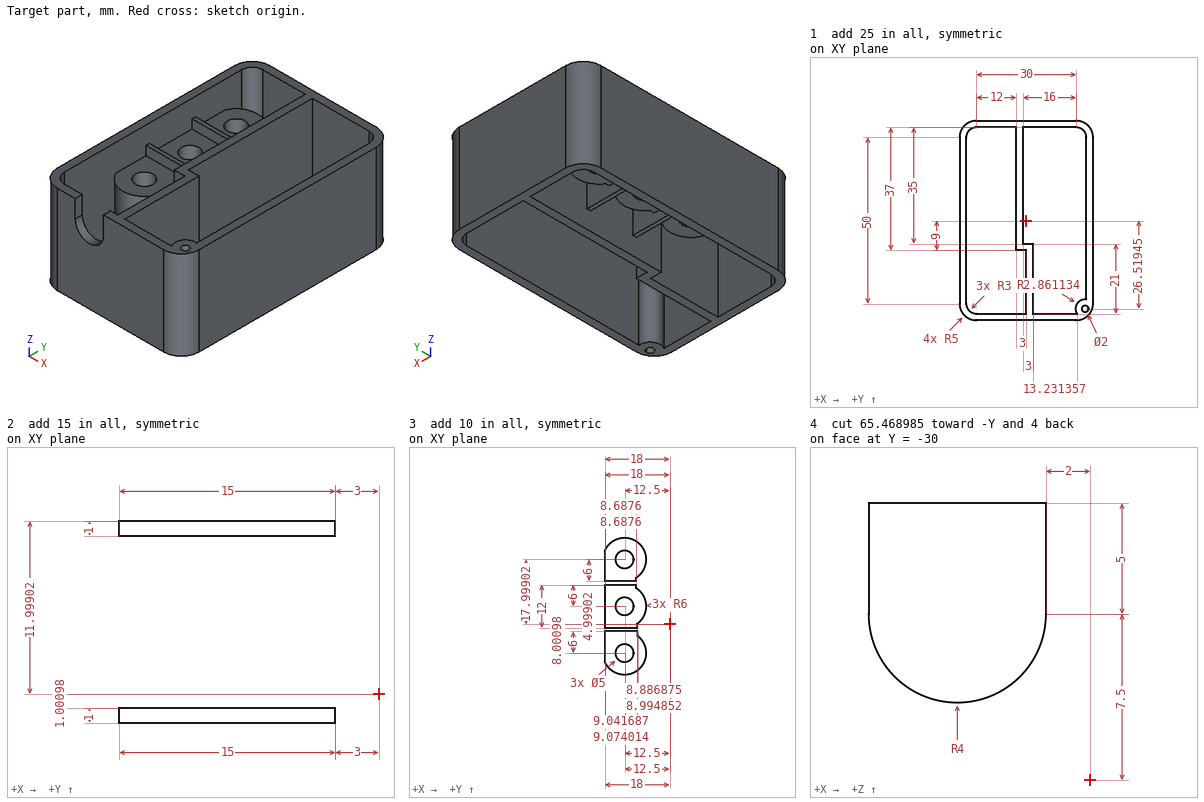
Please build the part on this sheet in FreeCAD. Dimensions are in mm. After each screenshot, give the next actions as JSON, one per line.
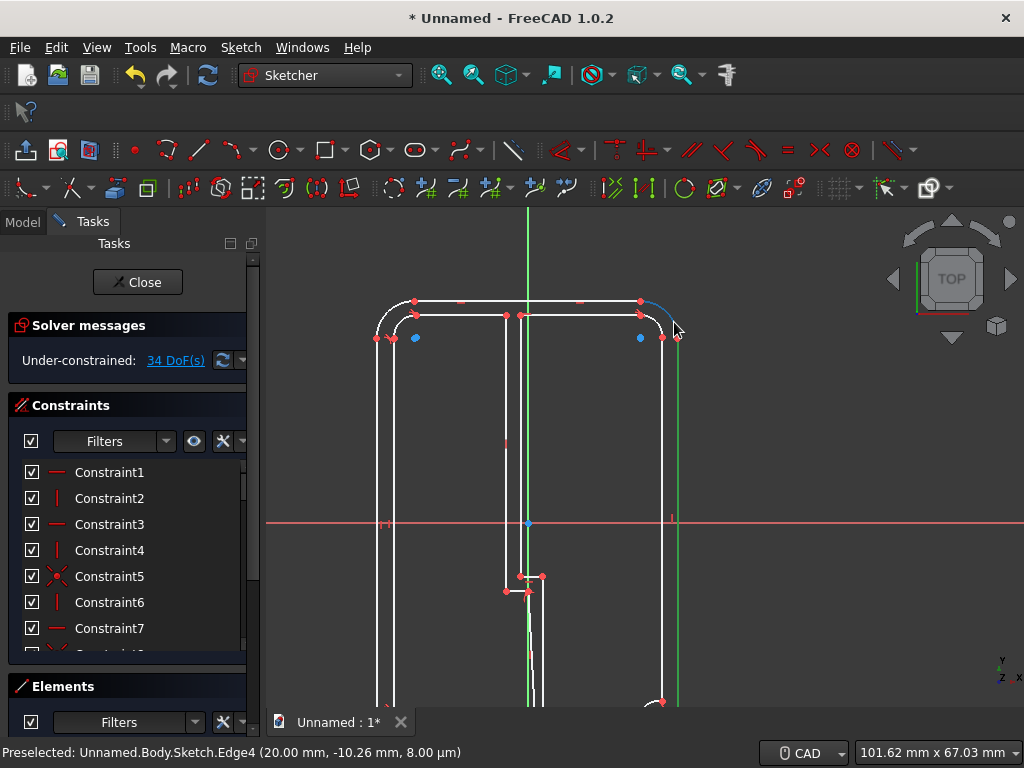
{"action": "left_click", "coordinate": [674, 322]}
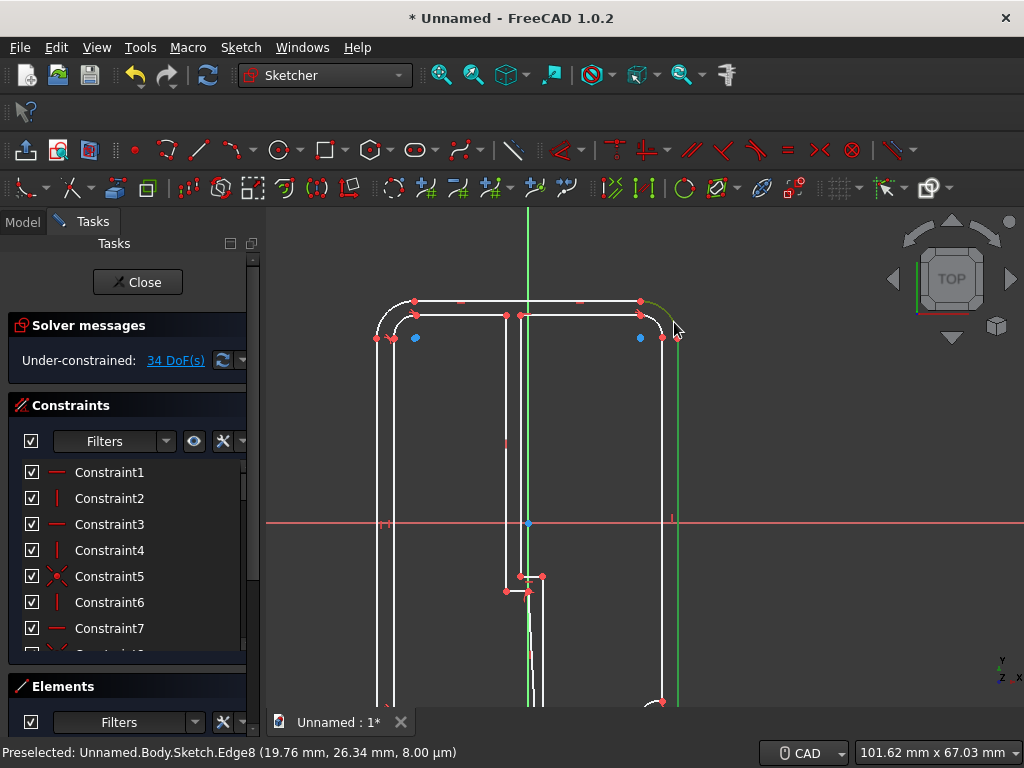
{"action": "left_click", "coordinate": [756, 150]}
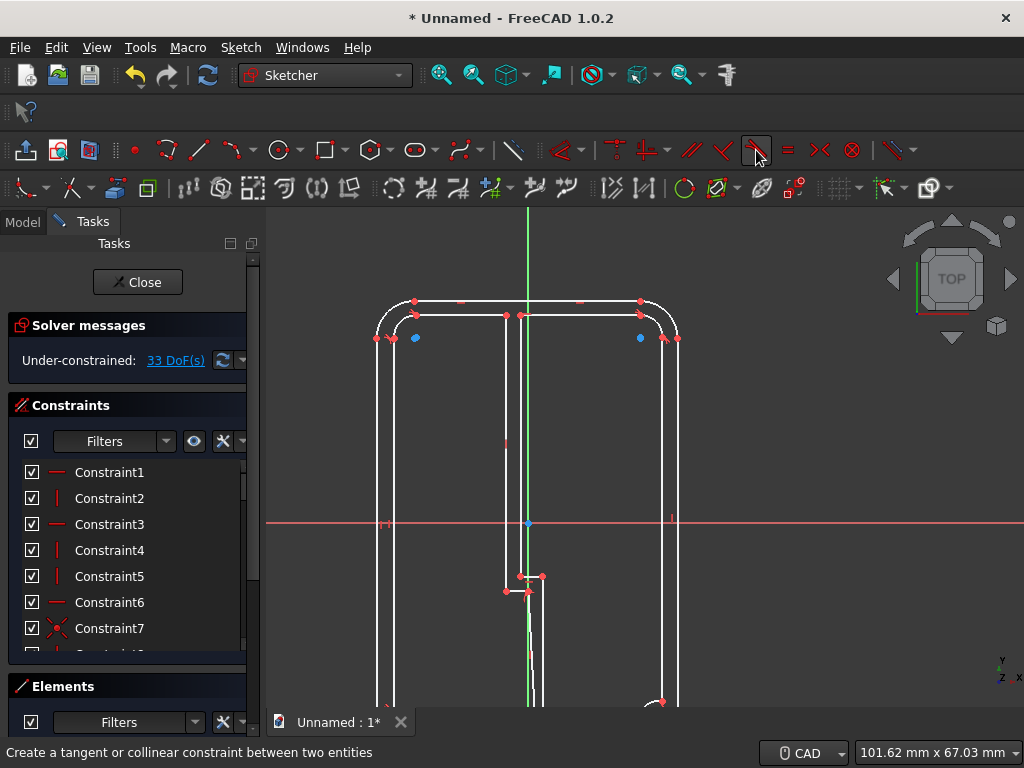
{"action": "left_click", "coordinate": [394, 599]}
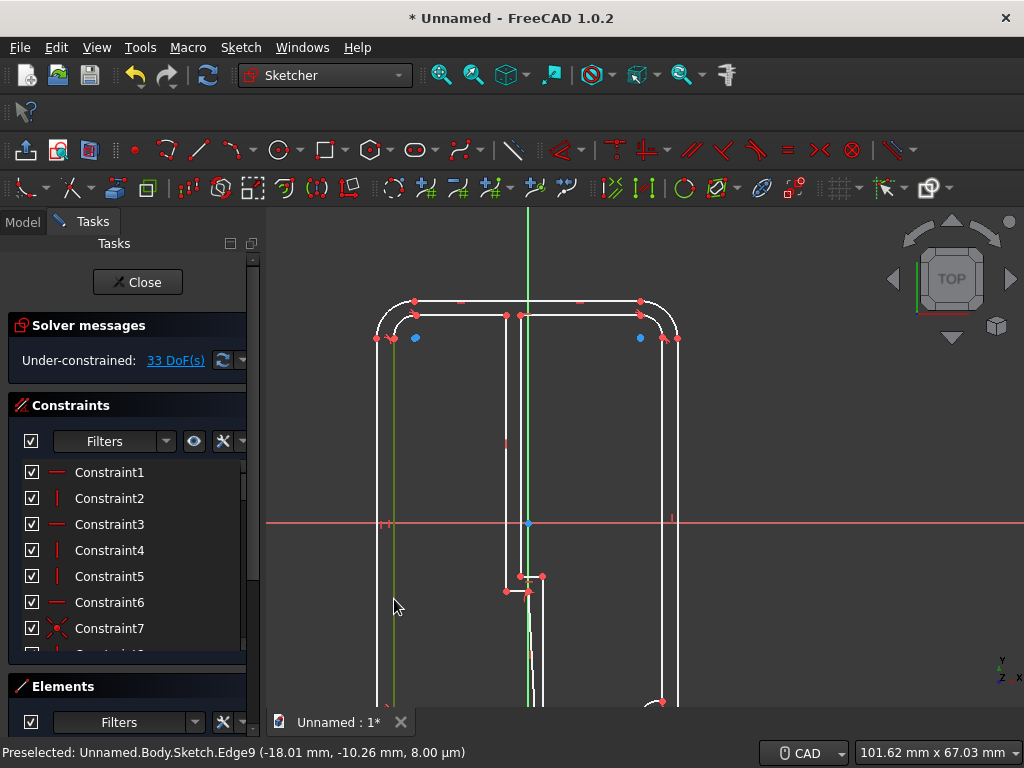
{"action": "scroll", "coordinate": [406, 318], "scroll_direction": "up", "scroll_amount": 2}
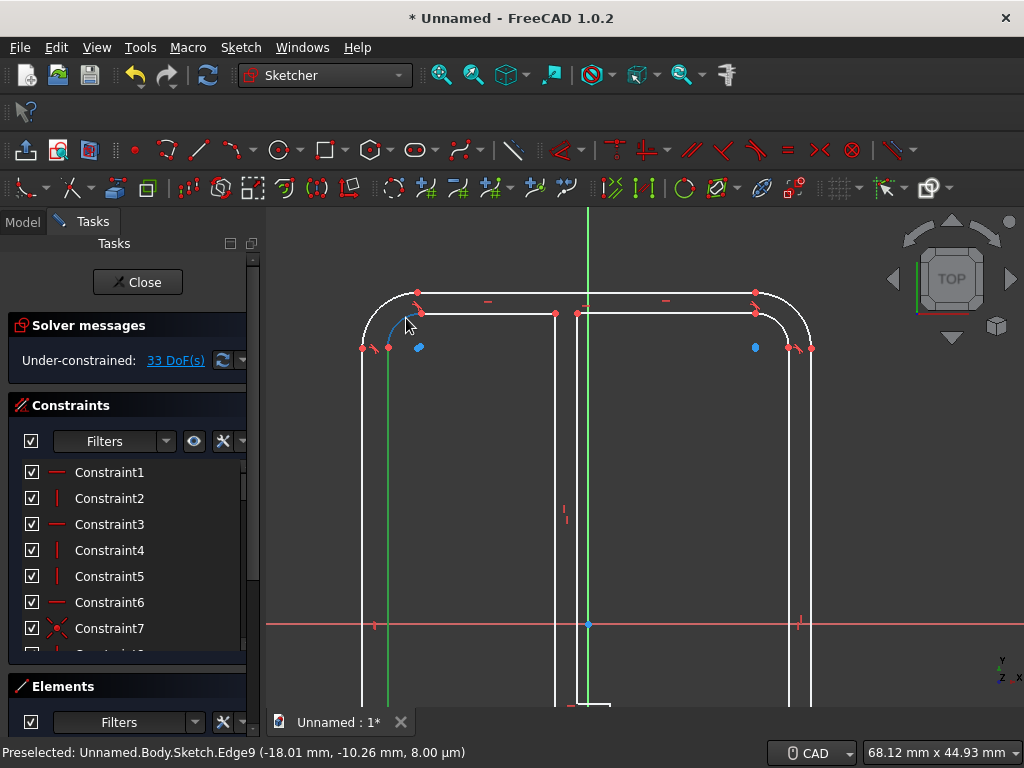
{"action": "left_click", "coordinate": [406, 317]}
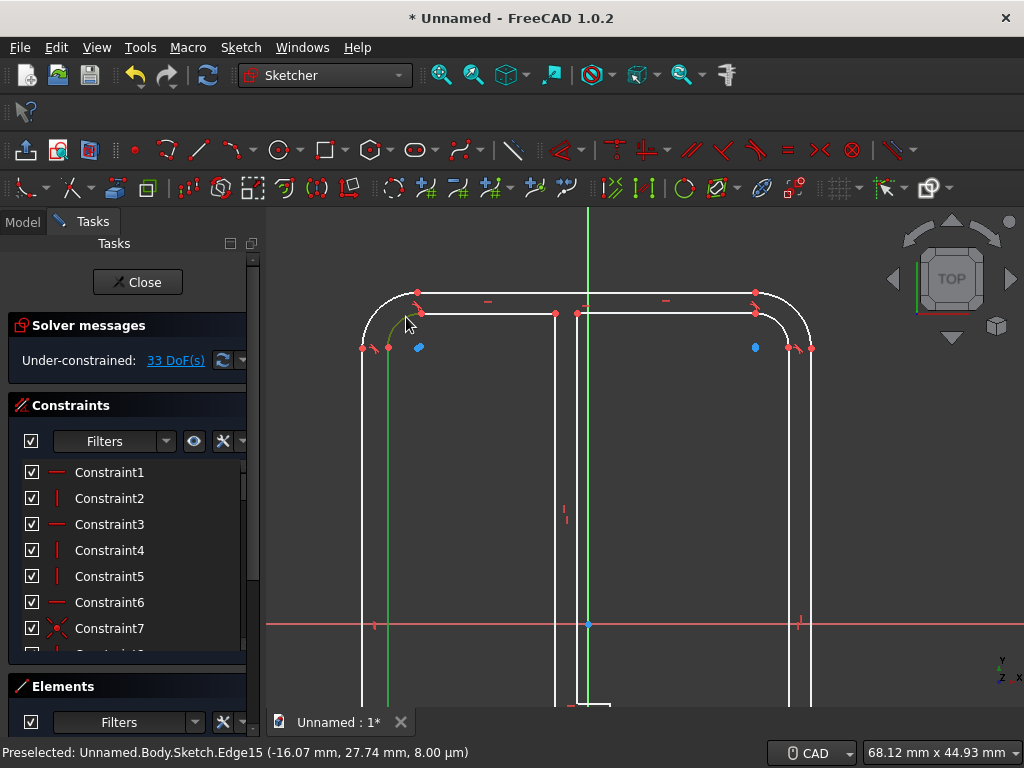
{"action": "left_click", "coordinate": [756, 150]}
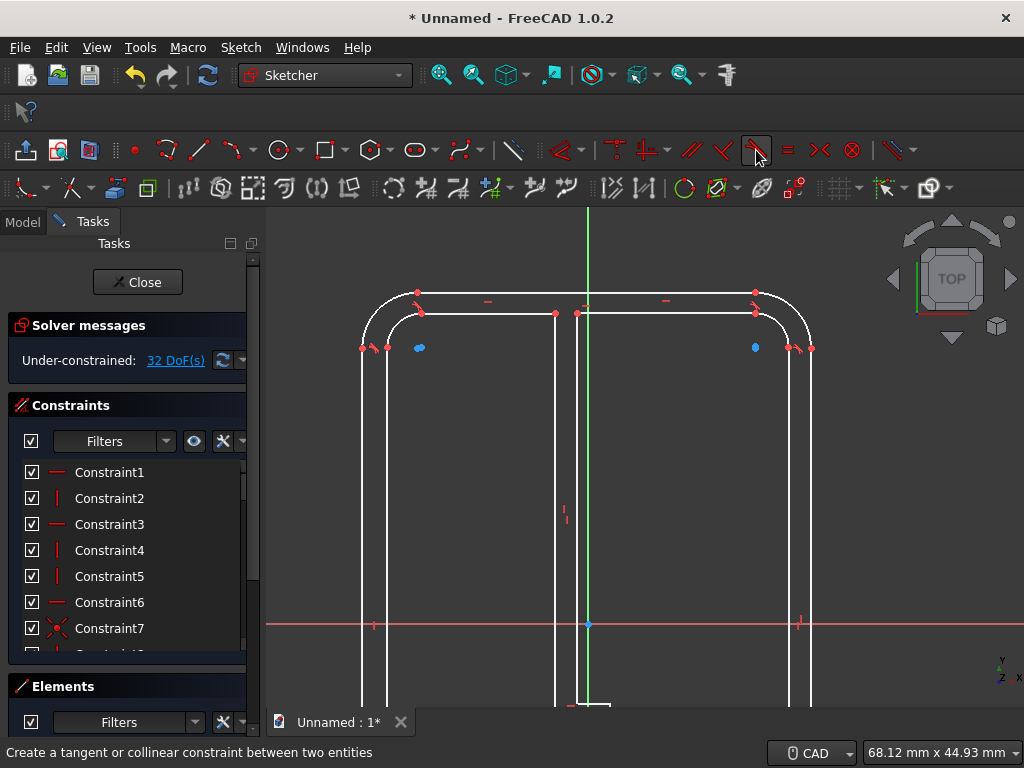
{"action": "left_click", "coordinate": [387, 515]}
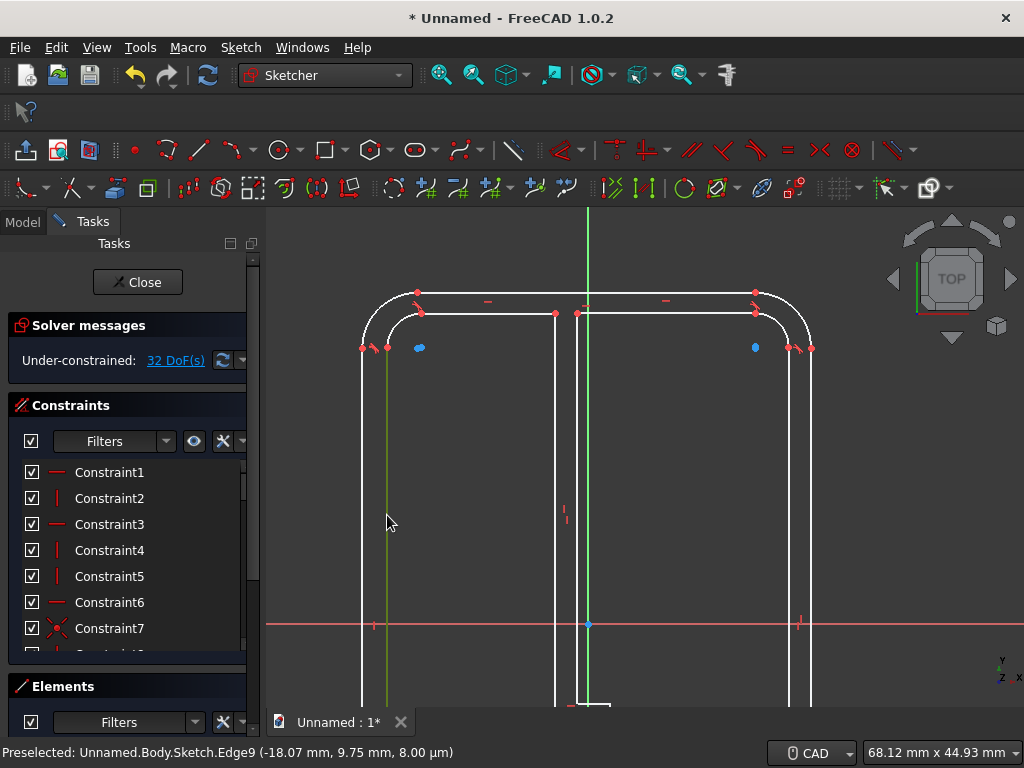
{"action": "scroll", "coordinate": [567, 320], "scroll_direction": "down", "scroll_amount": 4}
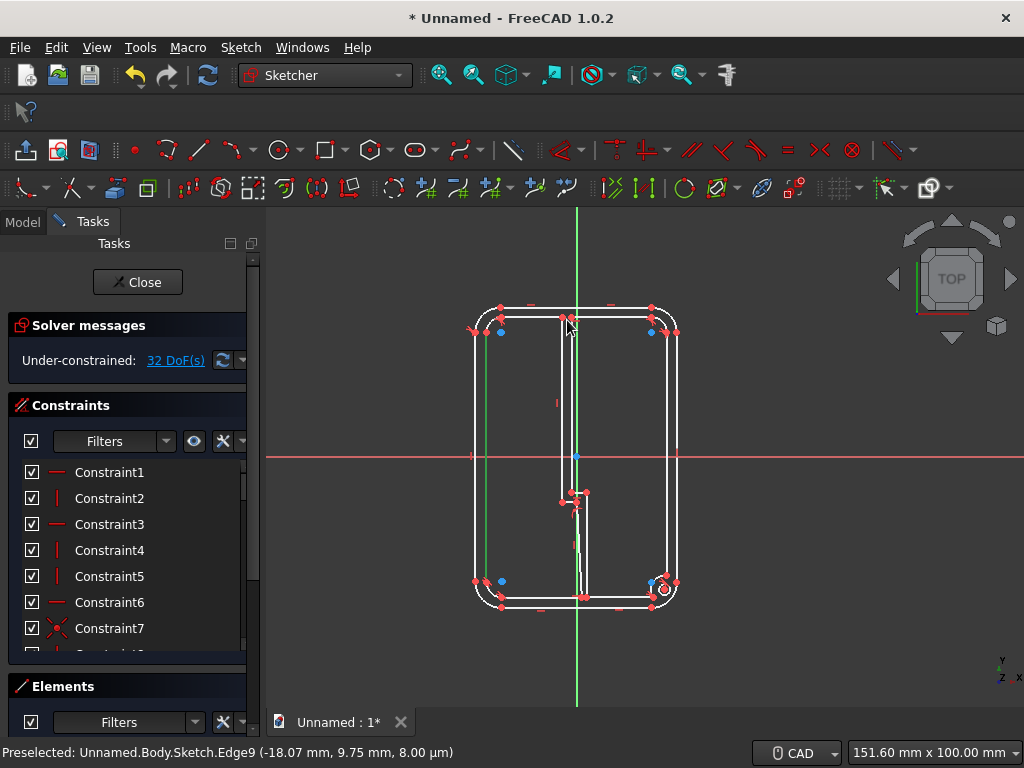
{"action": "scroll", "coordinate": [488, 589], "scroll_direction": "up", "scroll_amount": 4}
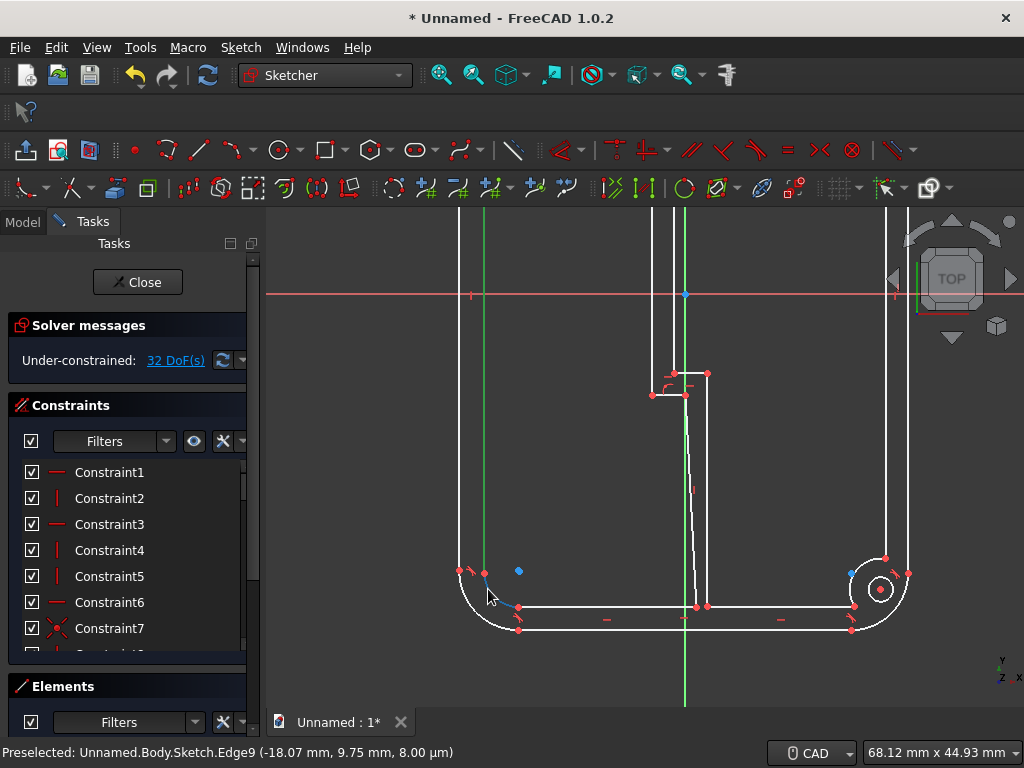
{"action": "left_click", "coordinate": [488, 588]}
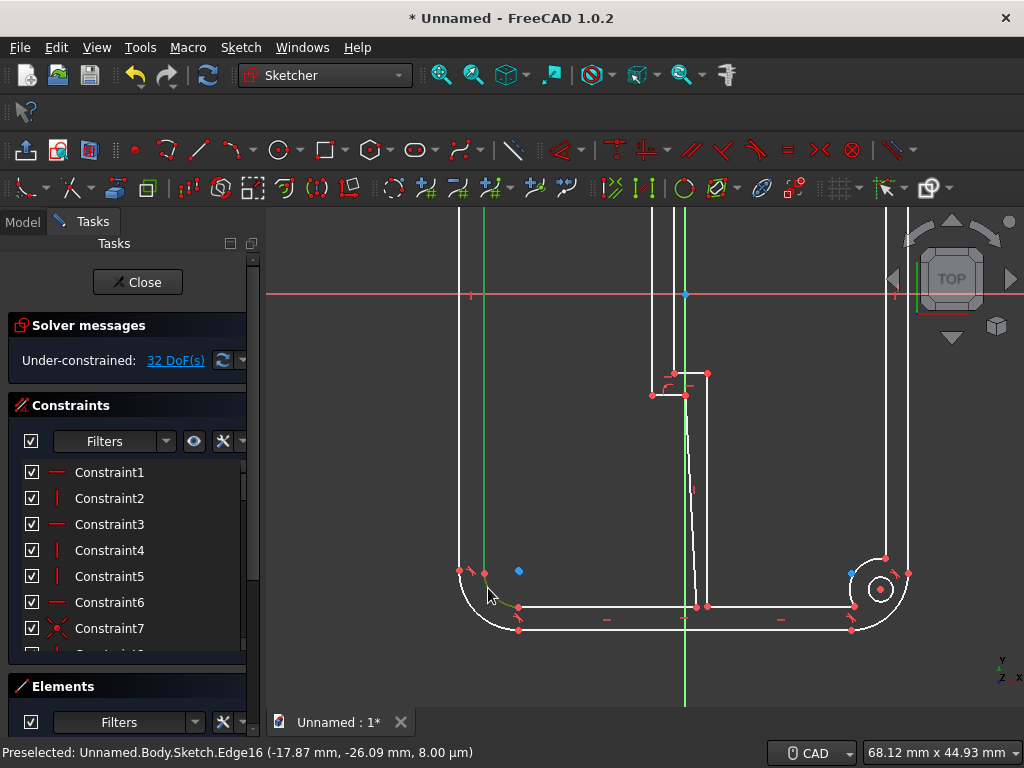
{"action": "left_click", "coordinate": [756, 150]}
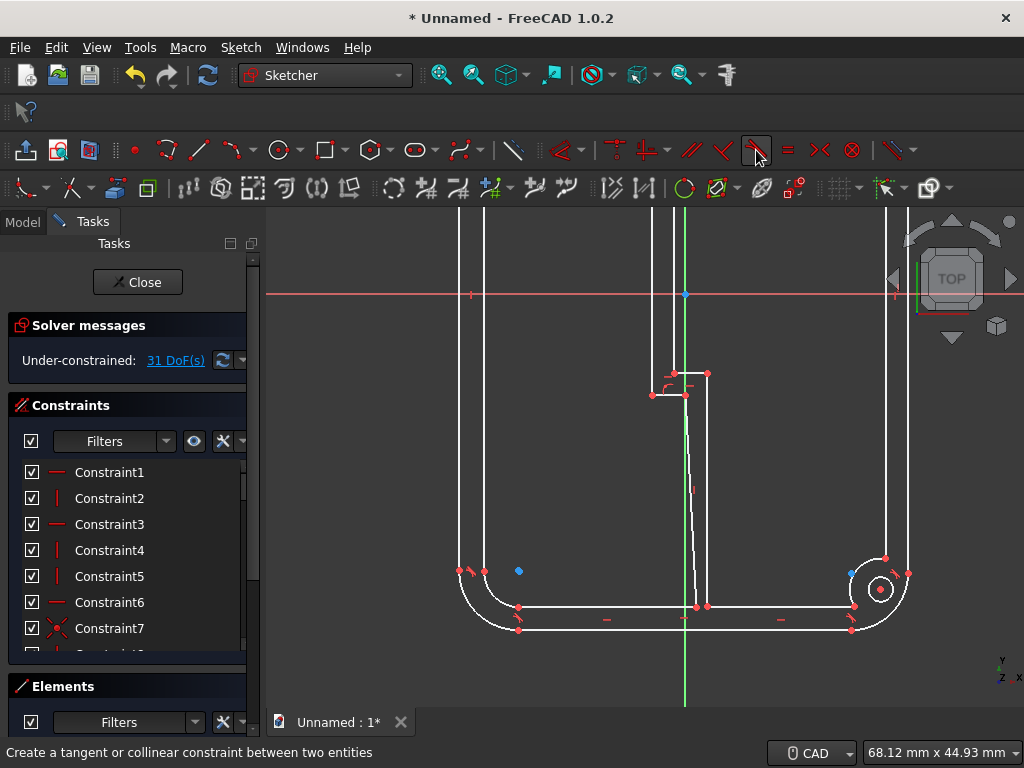
{"action": "scroll", "coordinate": [488, 590], "scroll_direction": "down", "scroll_amount": 4}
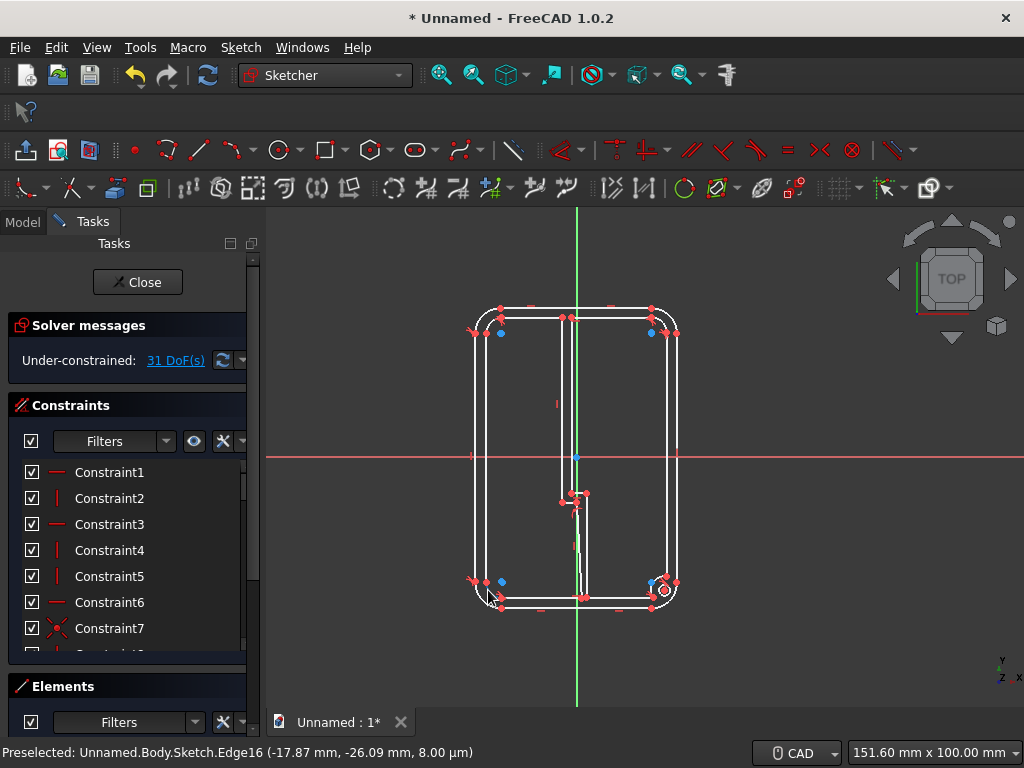
{"action": "scroll", "coordinate": [520, 318], "scroll_direction": "up", "scroll_amount": 2}